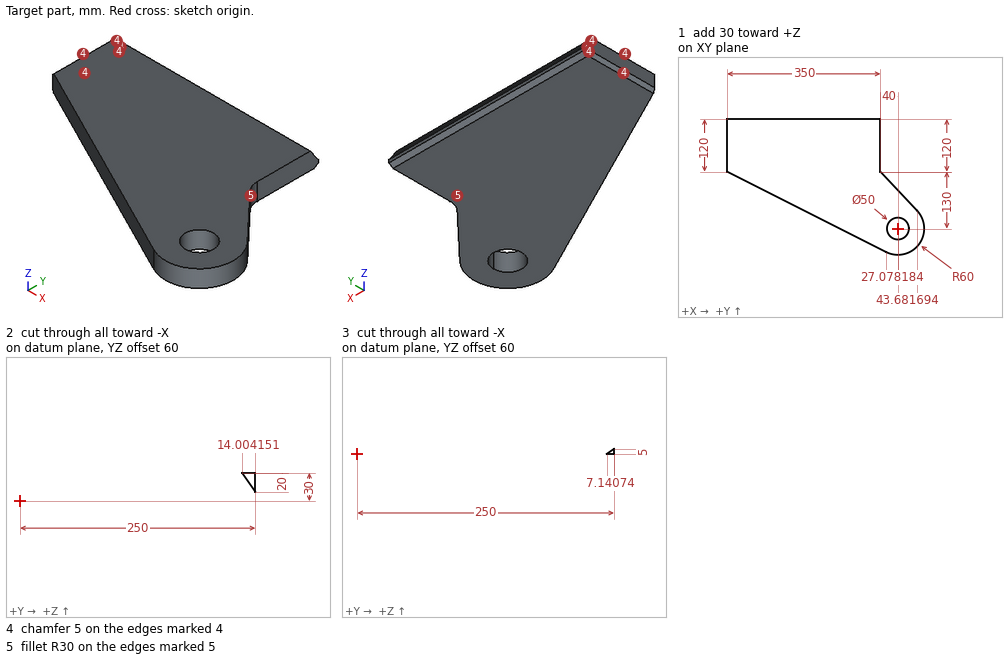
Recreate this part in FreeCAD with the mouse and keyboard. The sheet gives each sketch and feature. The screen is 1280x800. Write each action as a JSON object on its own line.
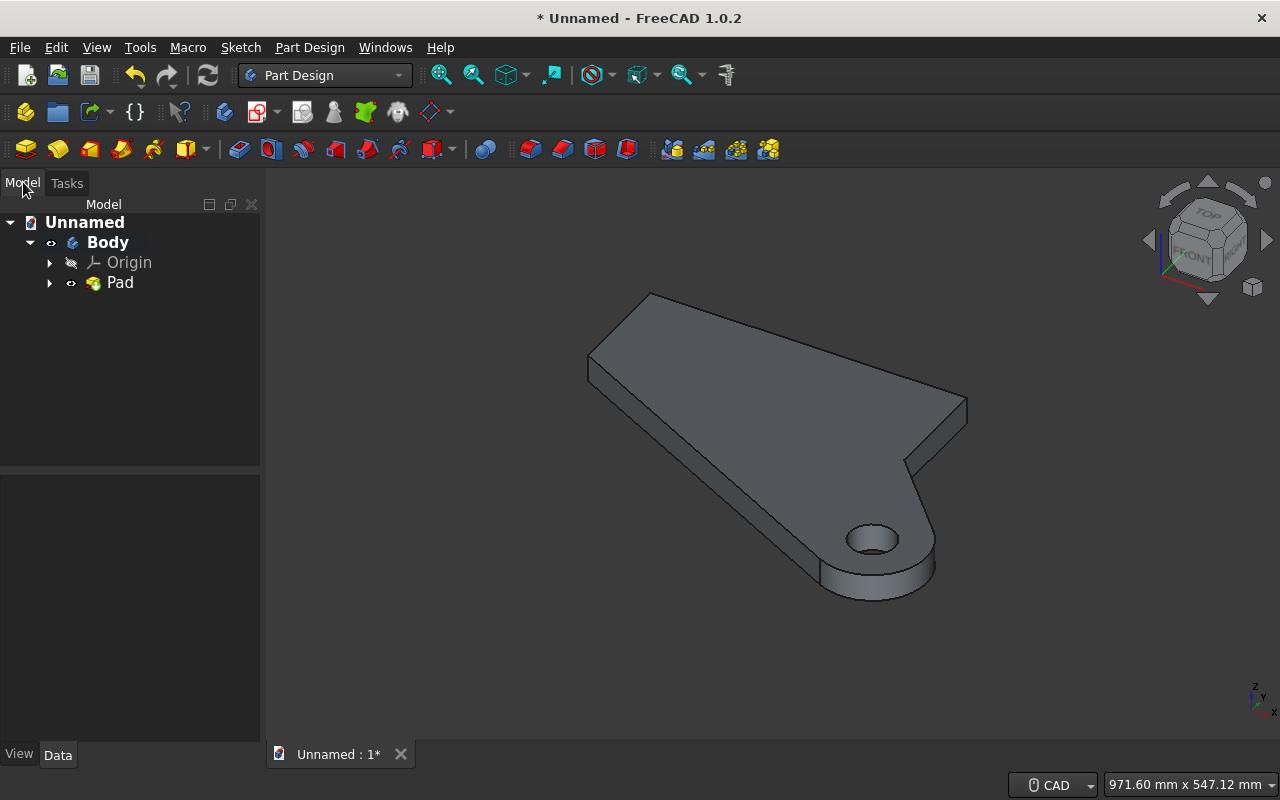
{"action": "left_click", "coordinate": [50, 263]}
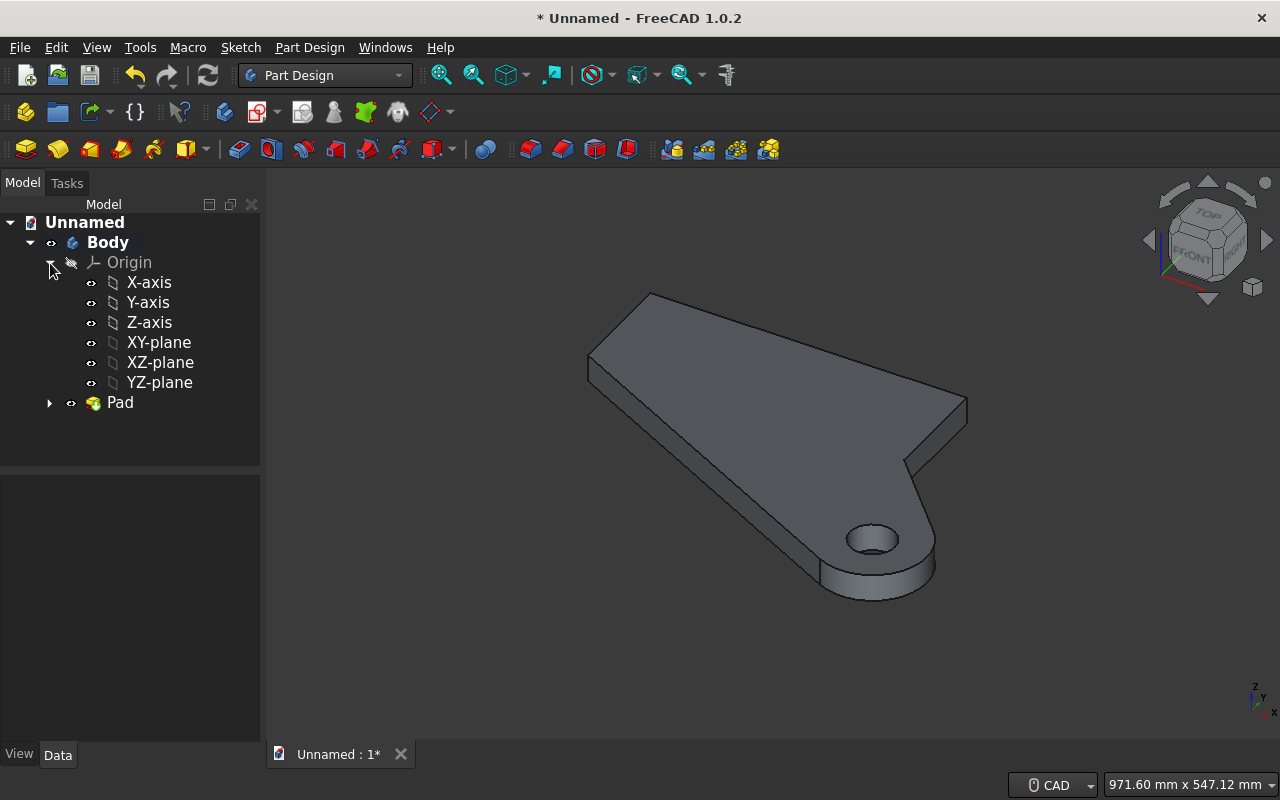
{"action": "left_click", "coordinate": [136, 383]}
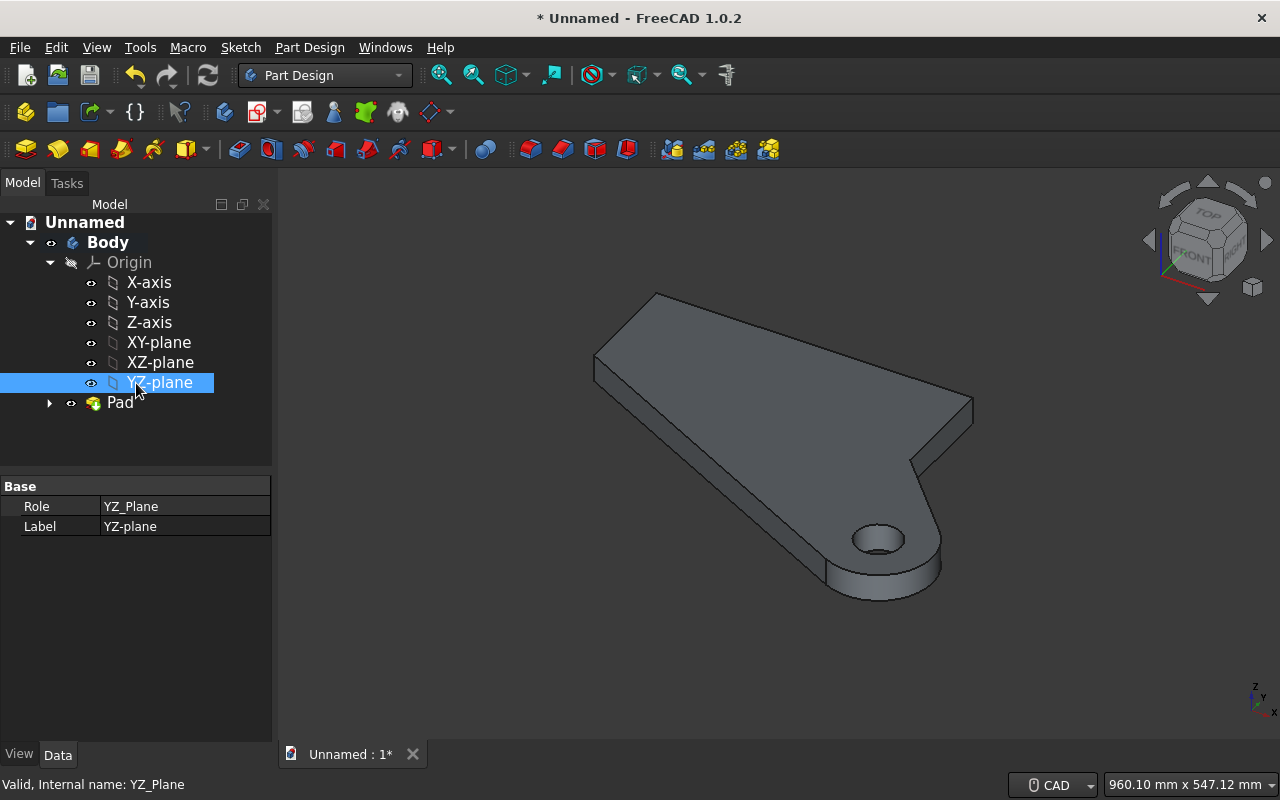
{"action": "left_click", "coordinate": [430, 112]}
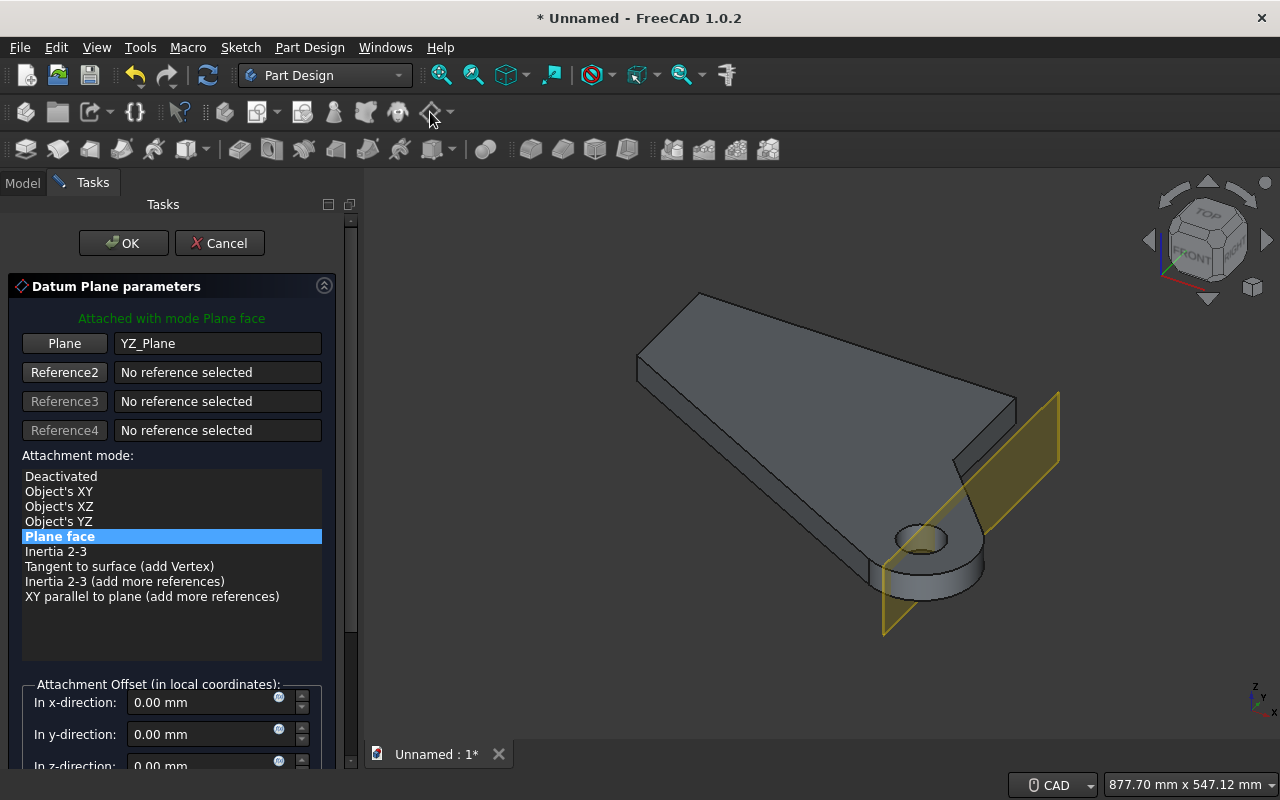
{"action": "scroll", "coordinate": [351, 491], "scroll_direction": "down", "scroll_amount": 2}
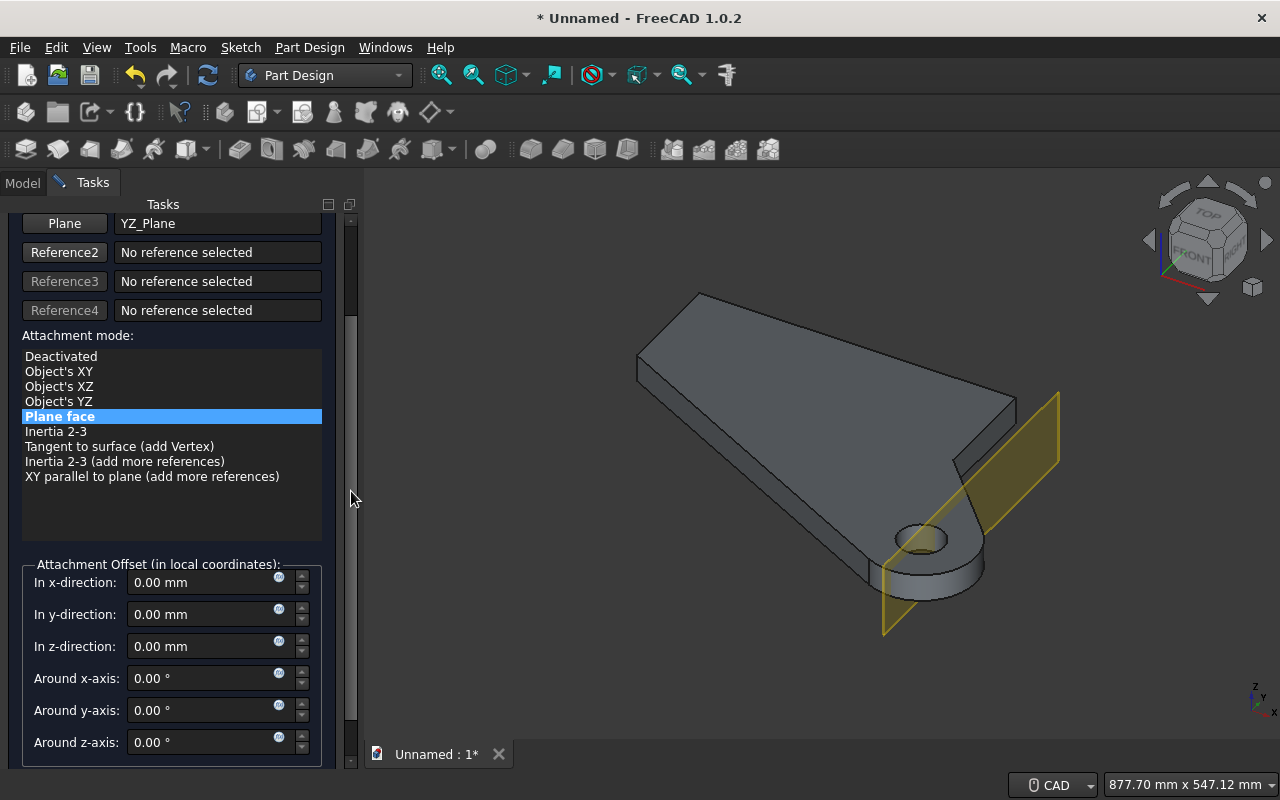
{"action": "triple_click", "coordinate": [210, 646]}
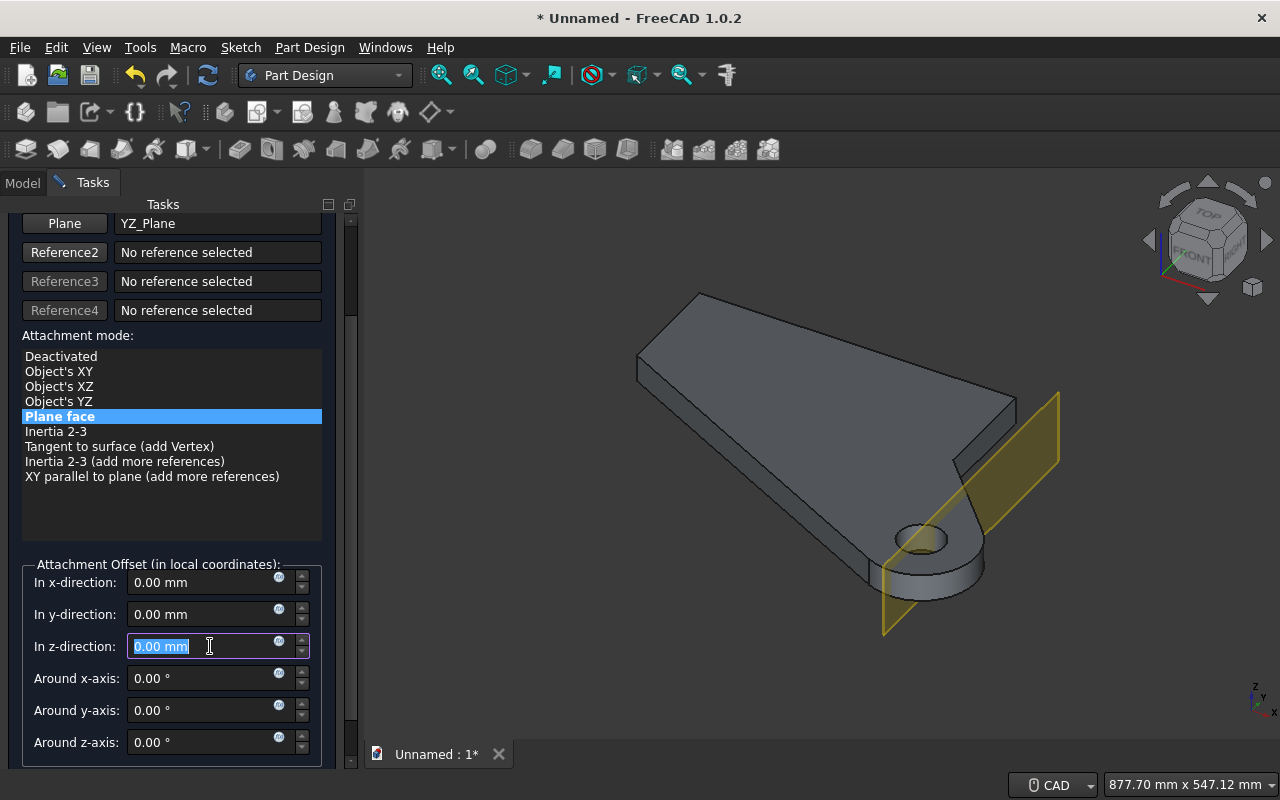
{"action": "type", "text": "60"}
{"action": "key", "text": "Tab"}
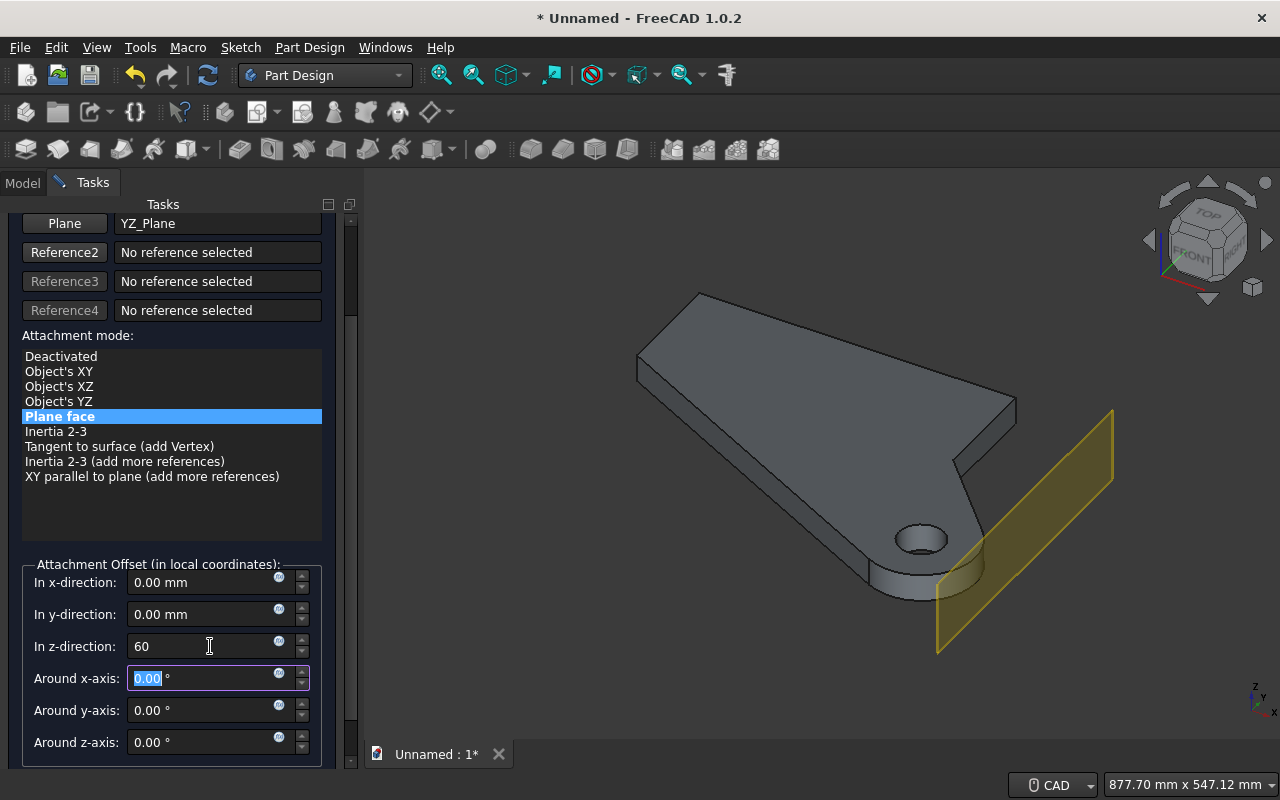
{"action": "scroll", "coordinate": [351, 491], "scroll_direction": "up", "scroll_amount": 3}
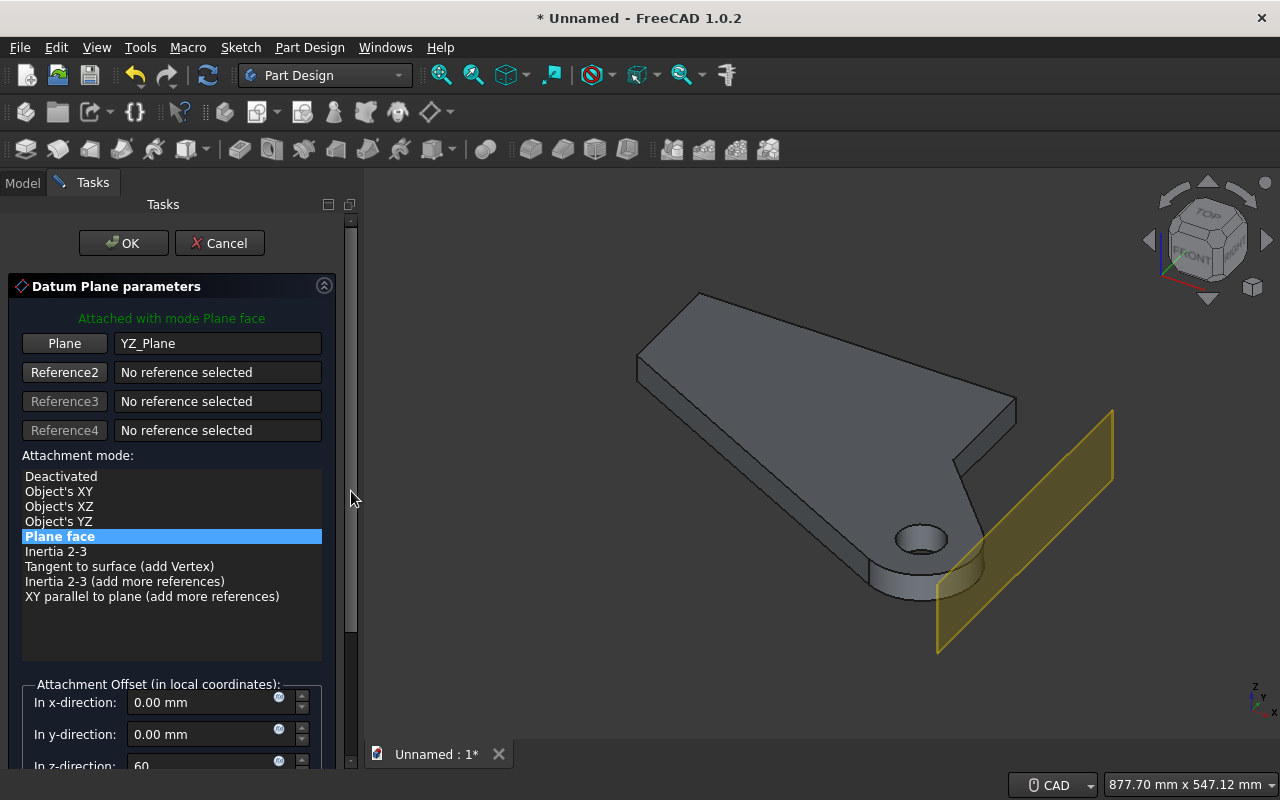
{"action": "left_click", "coordinate": [124, 243]}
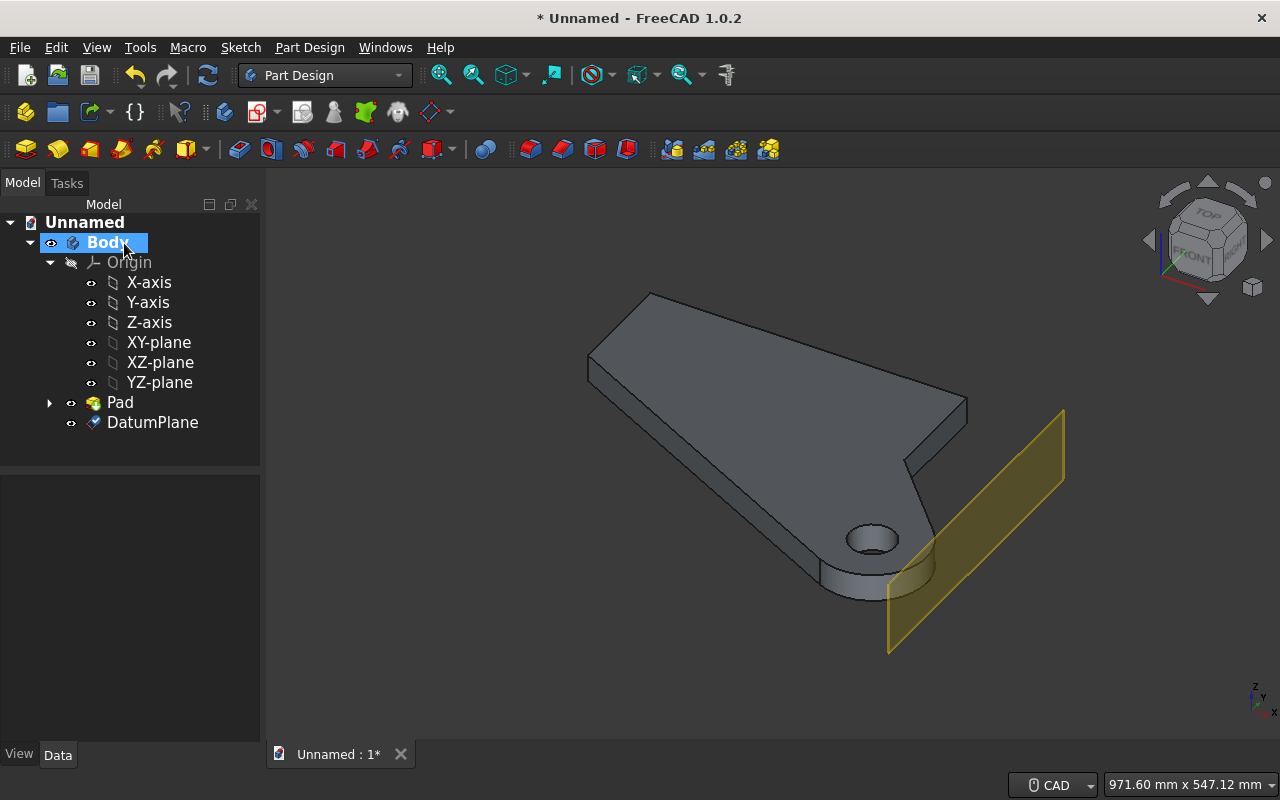
{"action": "left_click", "coordinate": [116, 423]}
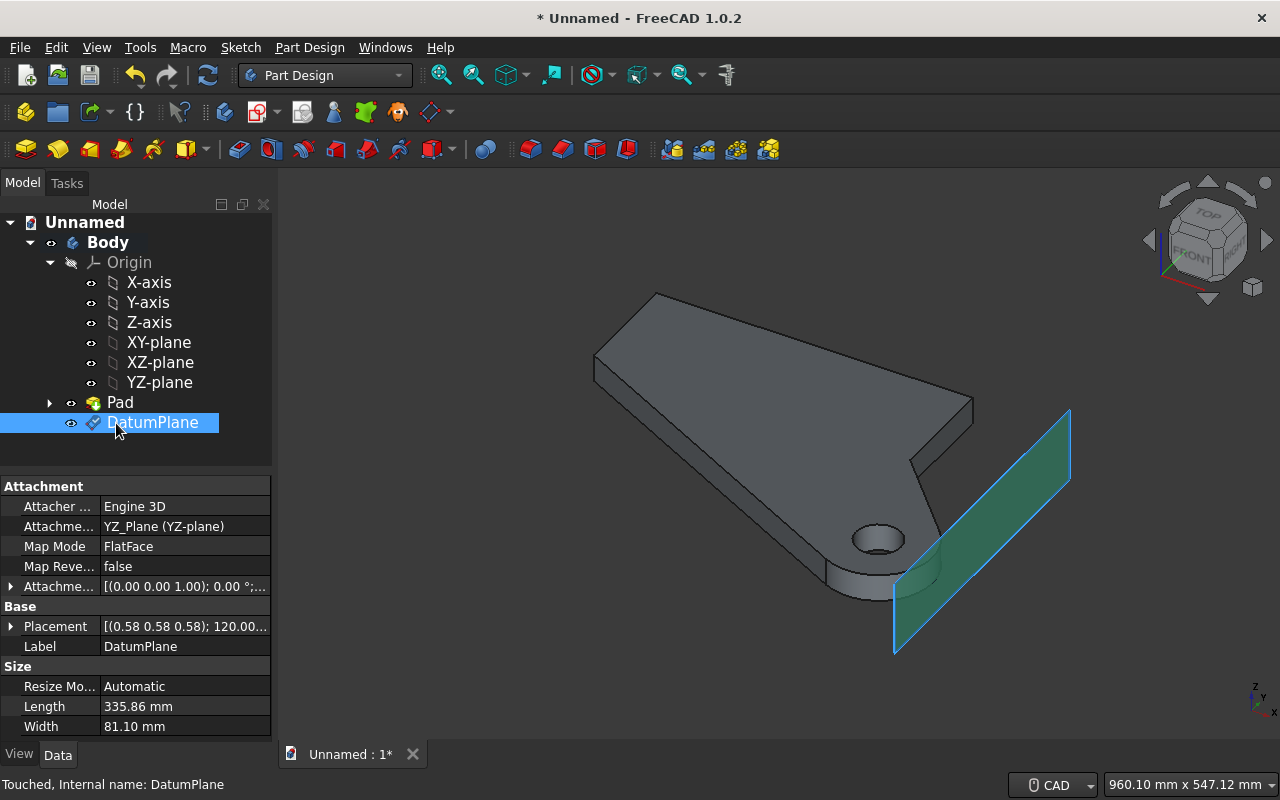
{"action": "left_click", "coordinate": [258, 112]}